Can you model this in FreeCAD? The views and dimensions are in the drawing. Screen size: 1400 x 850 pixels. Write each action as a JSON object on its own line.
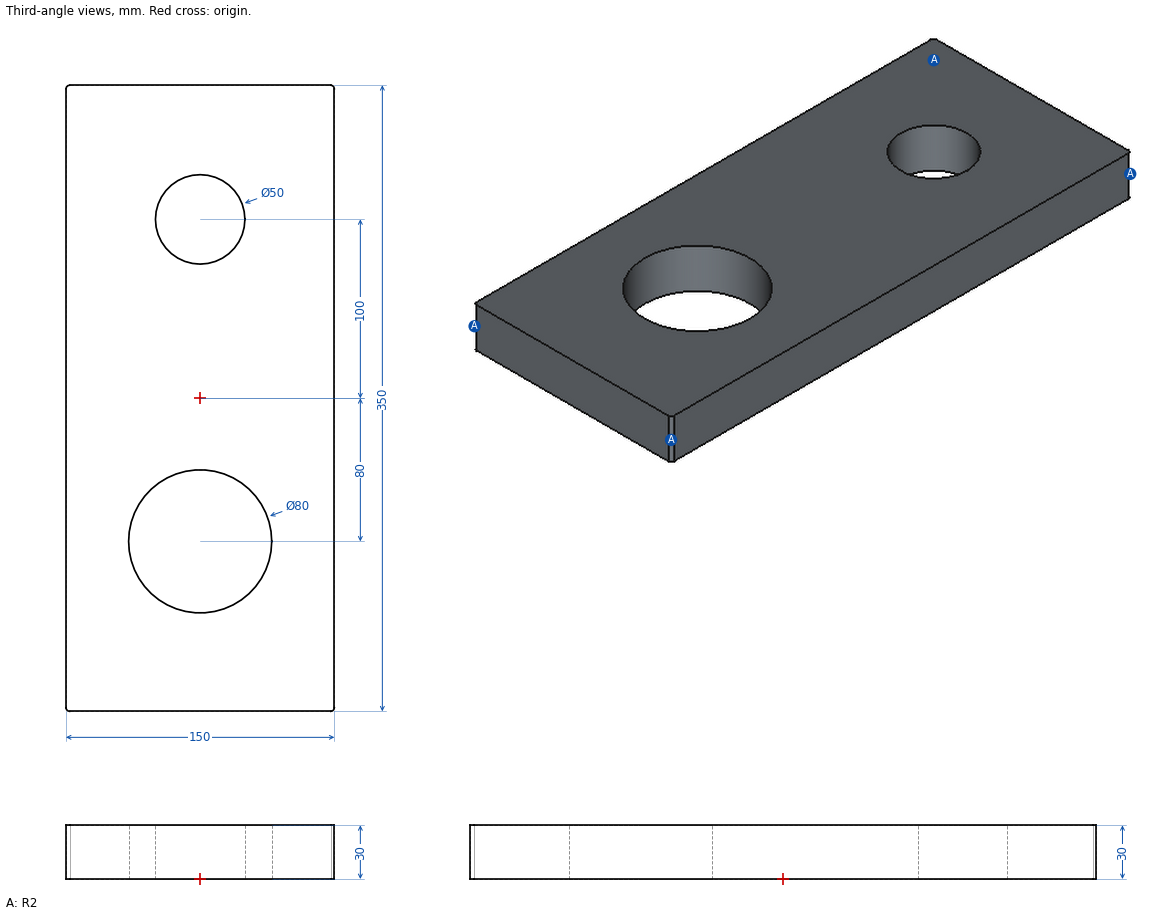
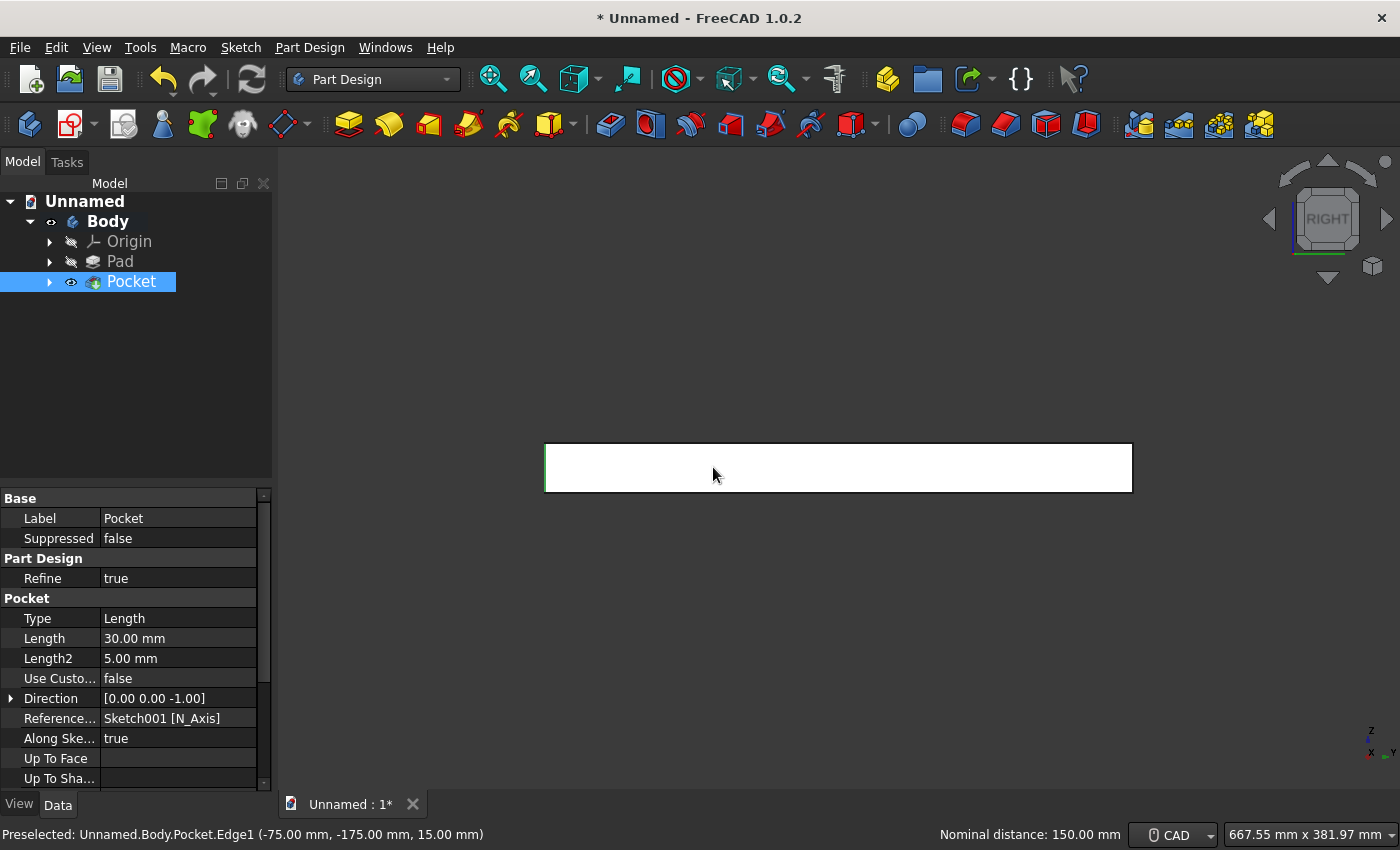
{"action": "left_click", "coordinate": [1133, 467], "text": "ctrl"}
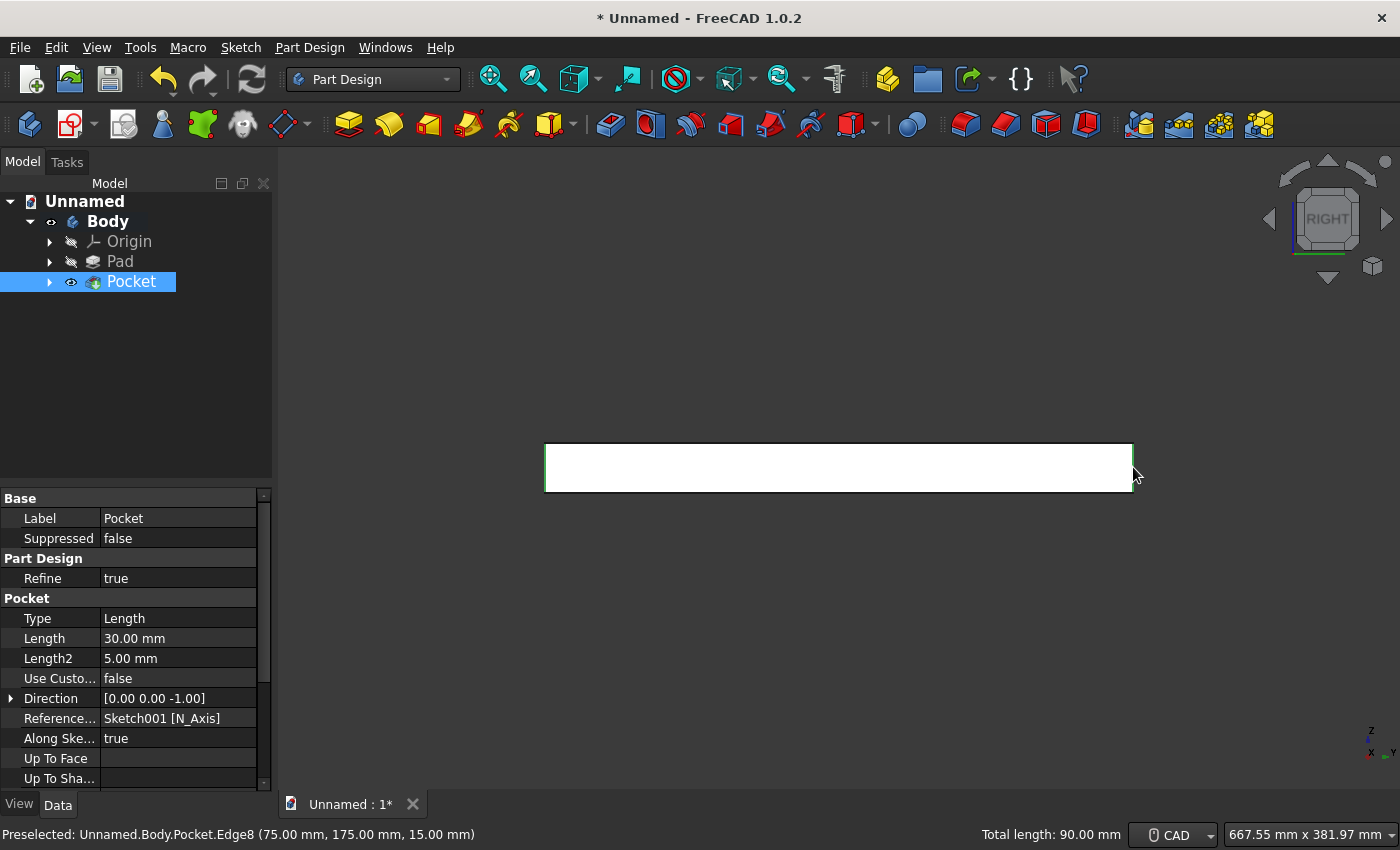
{"action": "key", "text": "5"}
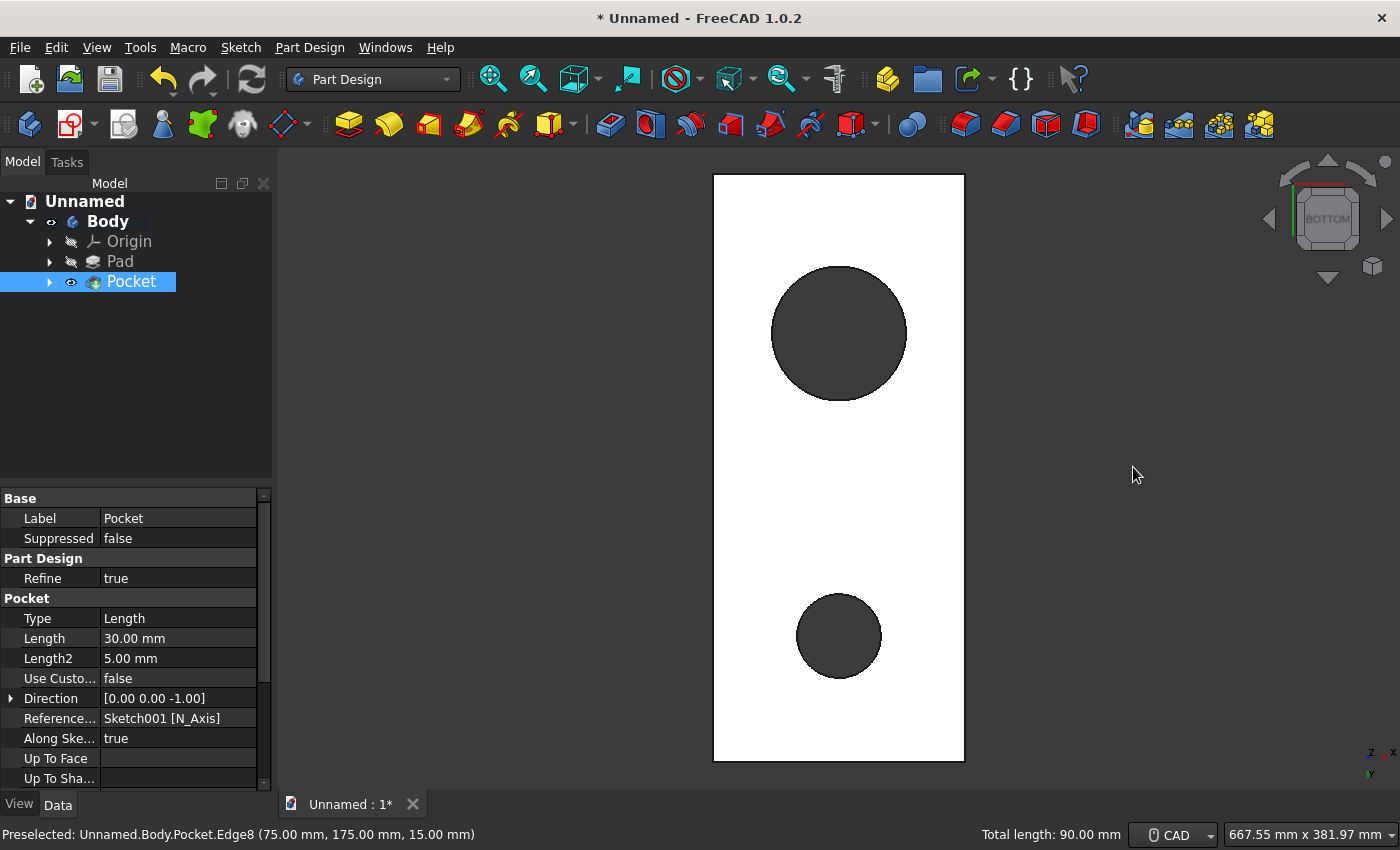
{"action": "key", "text": "4"}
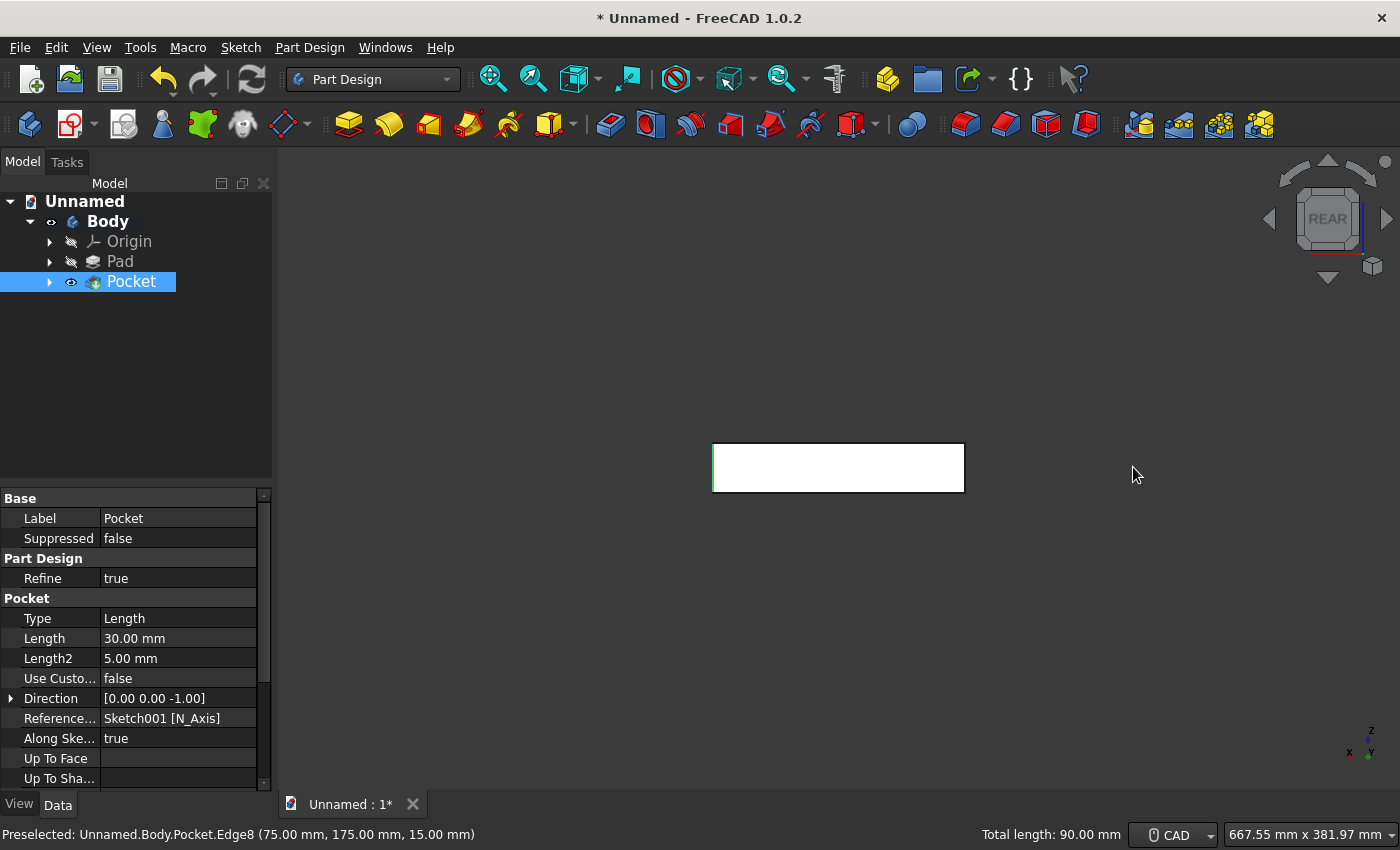
{"action": "left_click", "coordinate": [494, 80]}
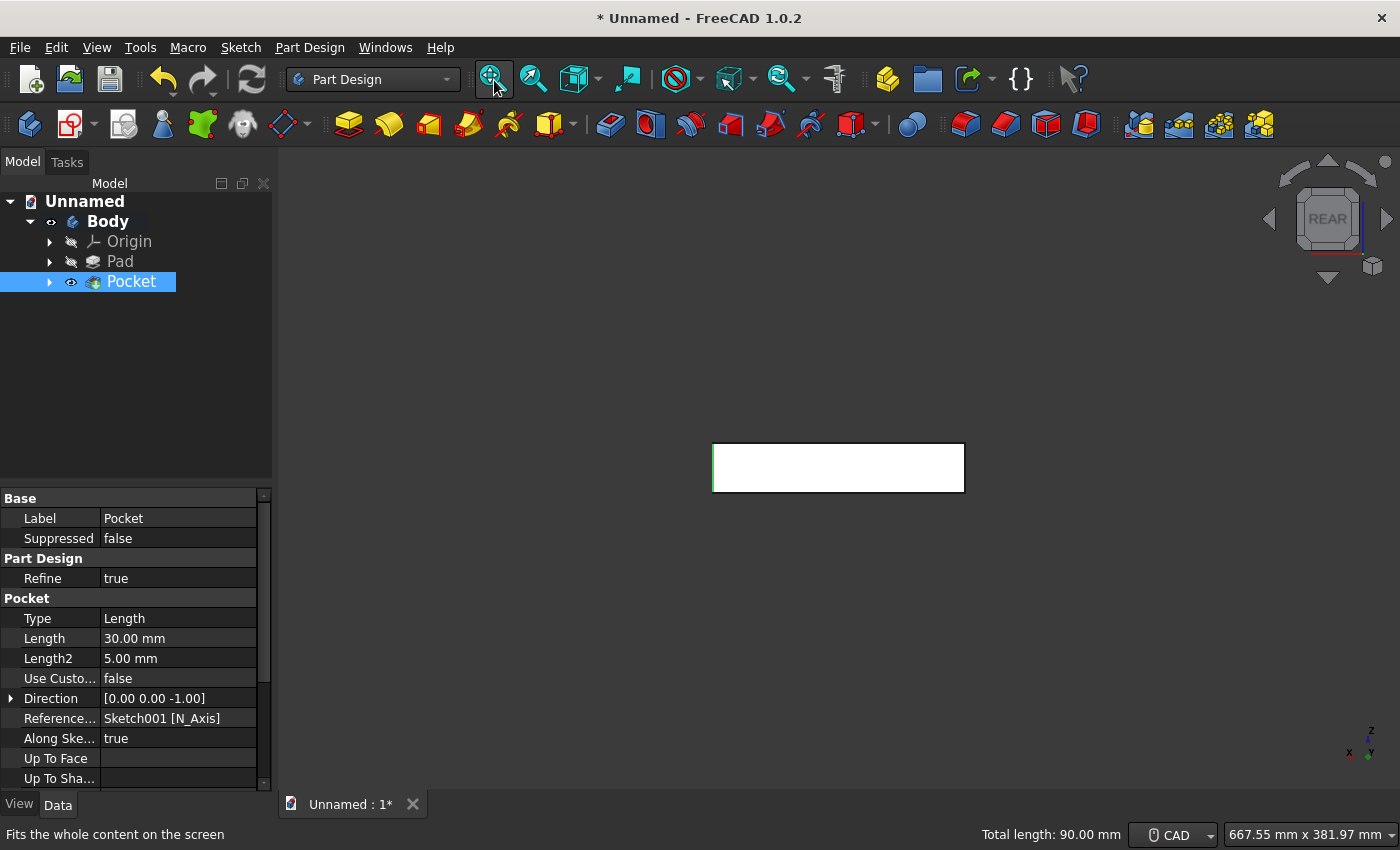
{"action": "left_click", "coordinate": [965, 467], "text": "ctrl"}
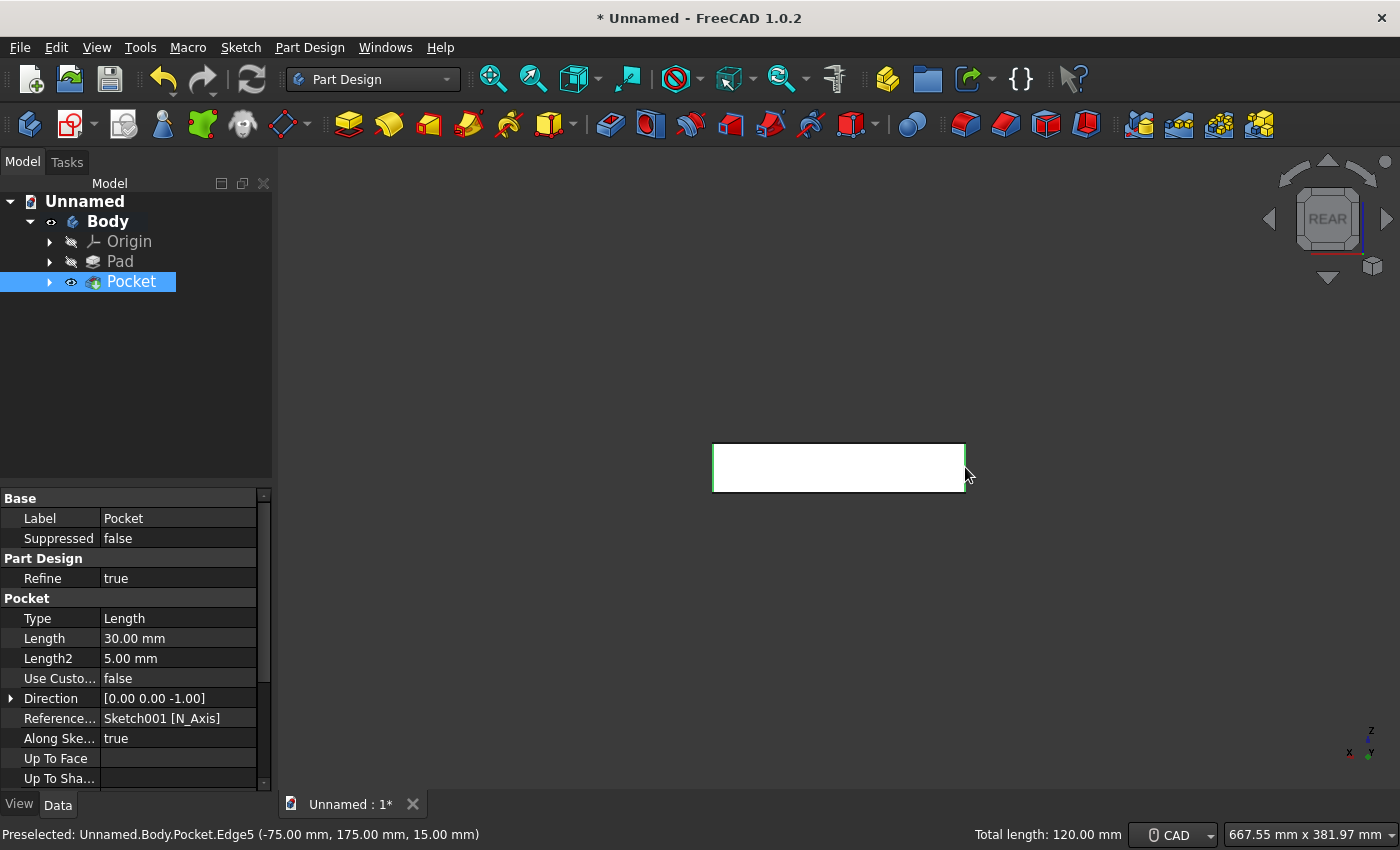
{"action": "left_click", "coordinate": [966, 124]}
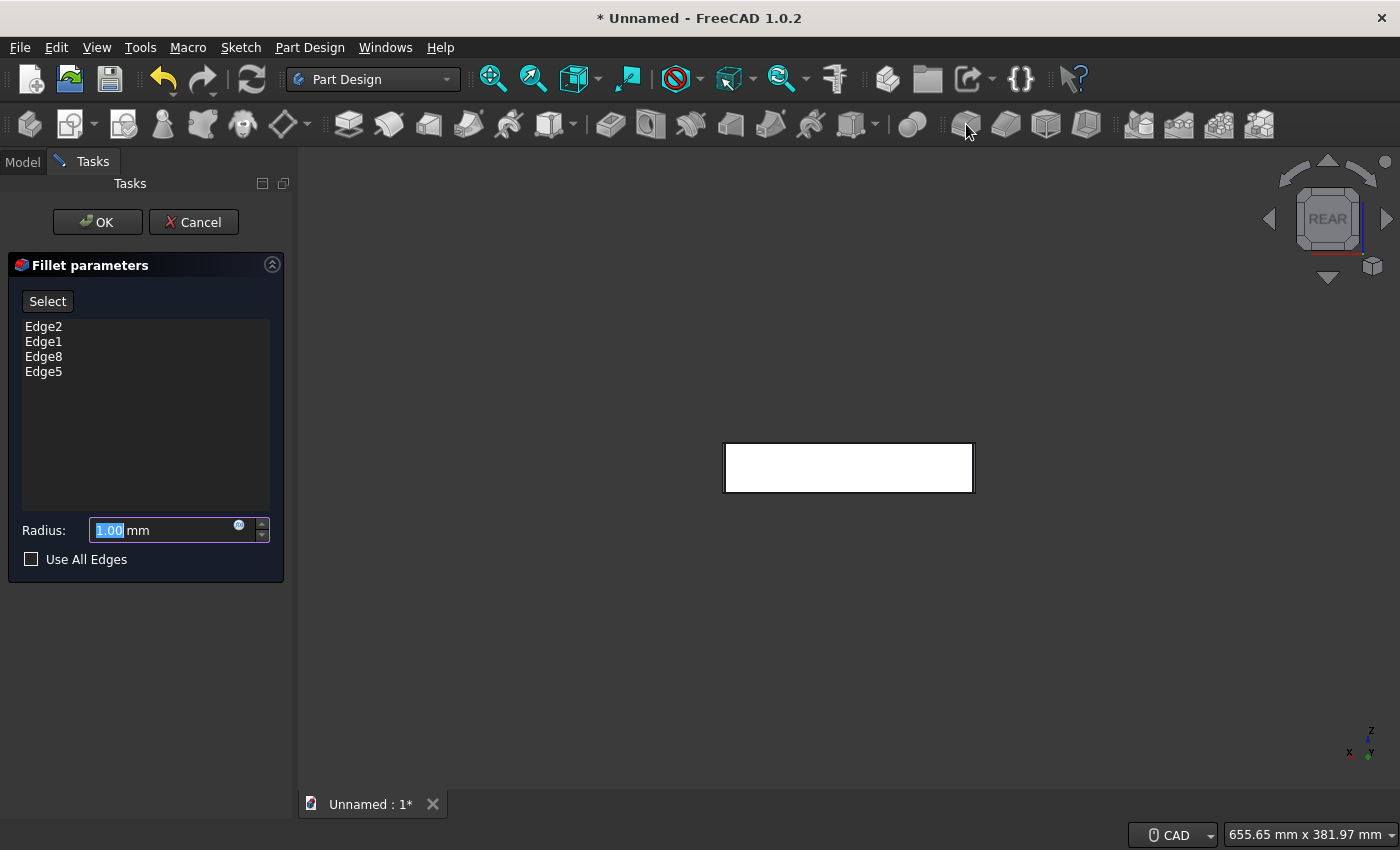
{"action": "type", "text": "2"}
{"action": "key", "text": "Tab"}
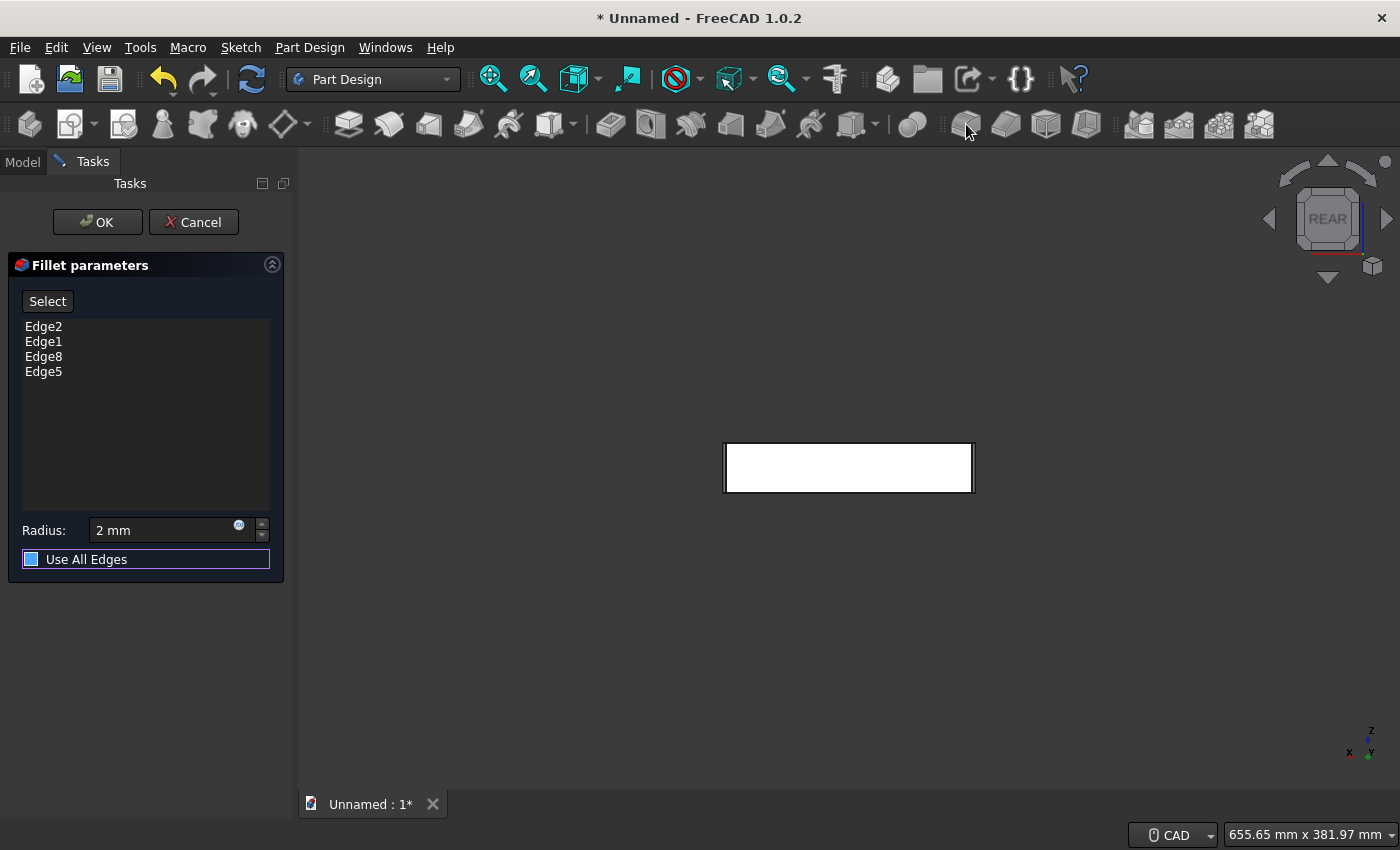
{"action": "left_click", "coordinate": [98, 222]}